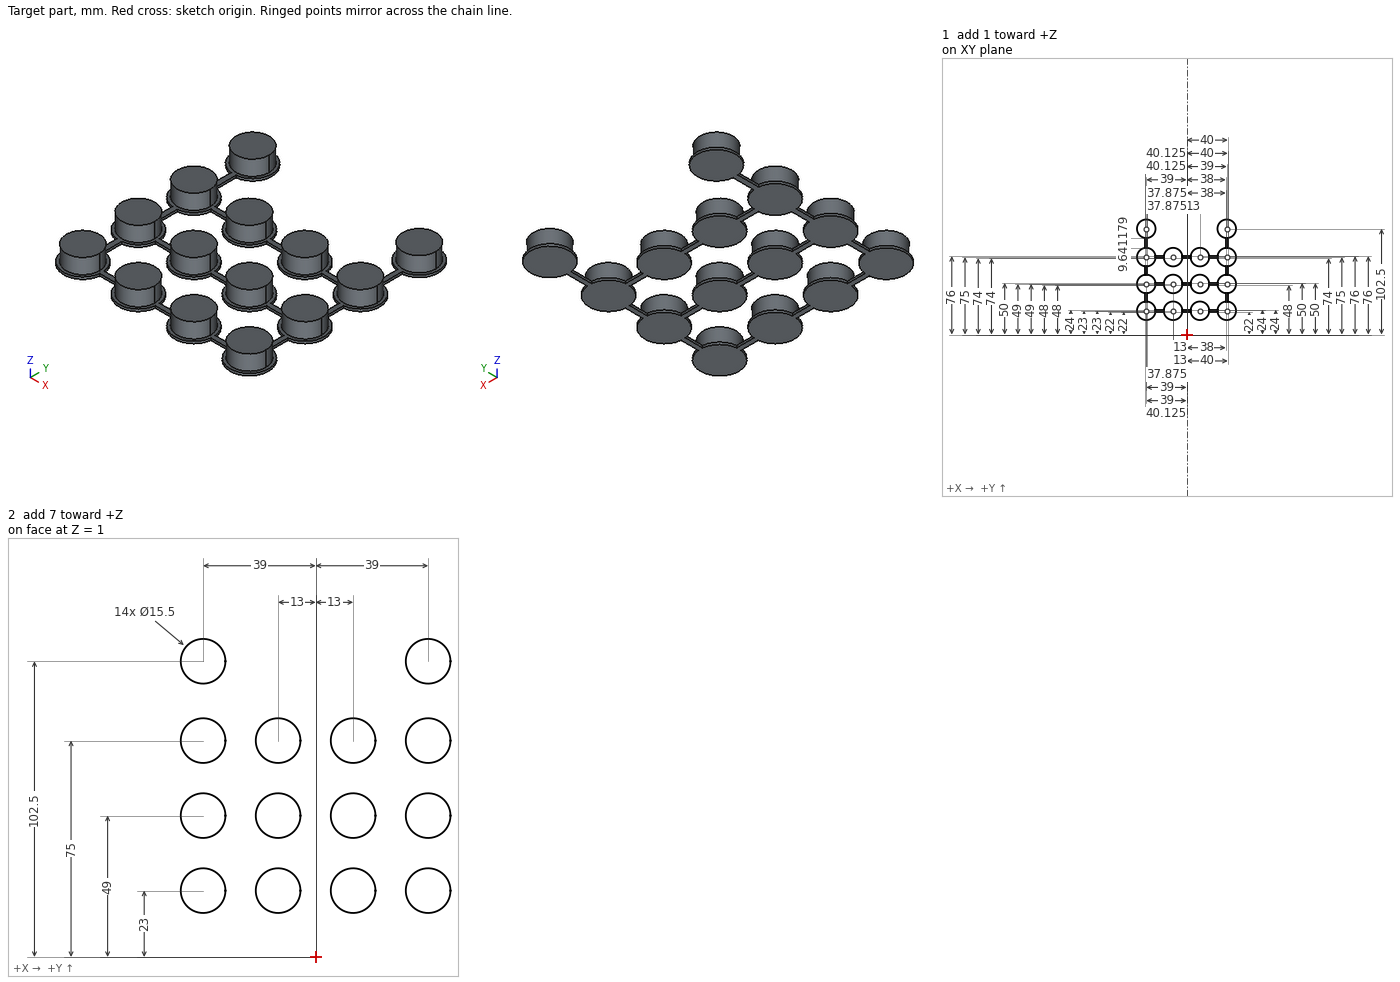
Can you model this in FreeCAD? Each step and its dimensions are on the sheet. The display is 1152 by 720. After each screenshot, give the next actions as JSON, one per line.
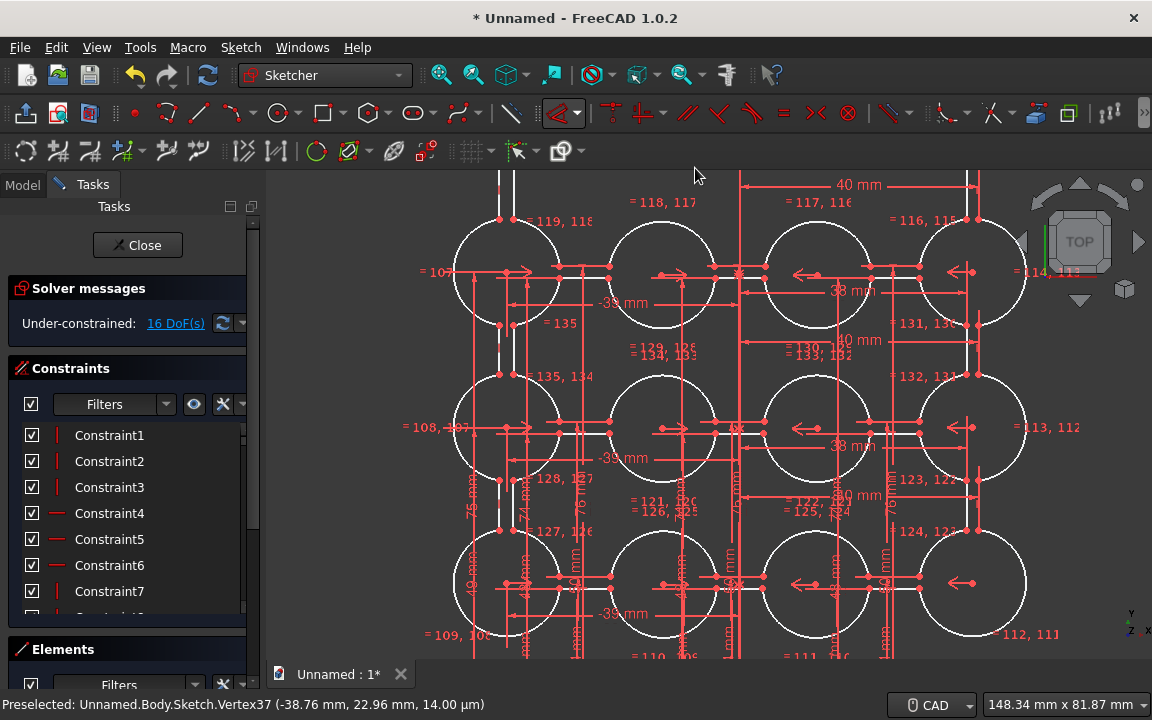
{"action": "left_click", "coordinate": [507, 583]}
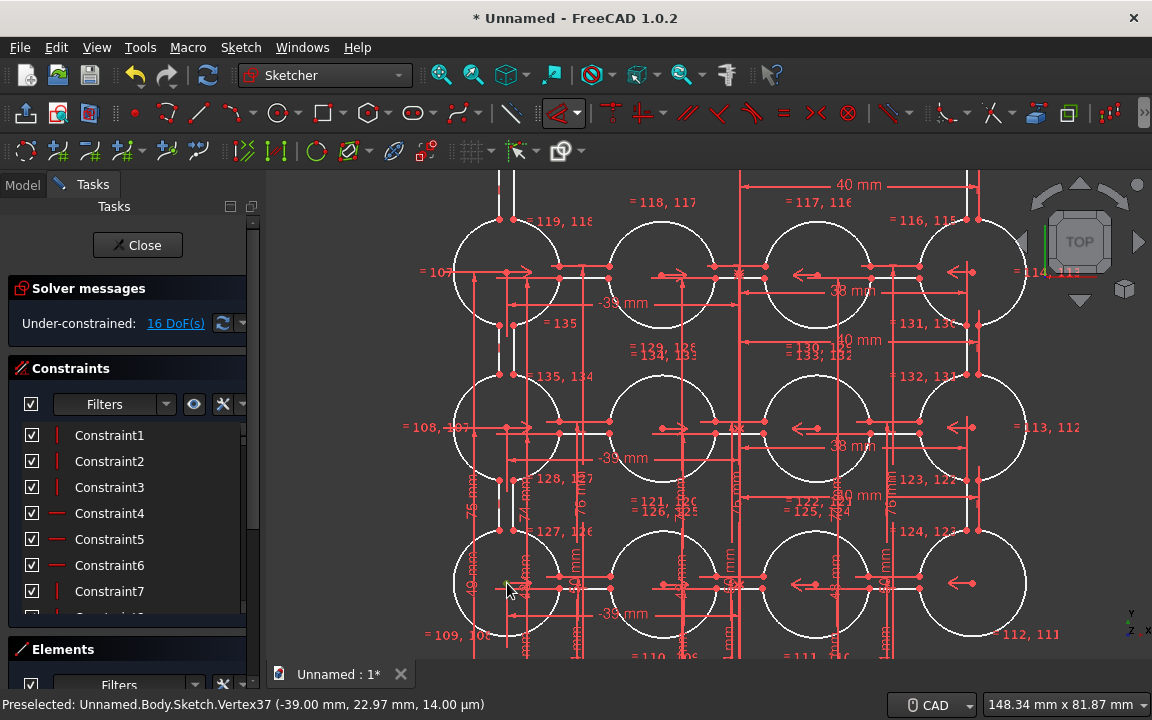
{"action": "key", "text": "i"}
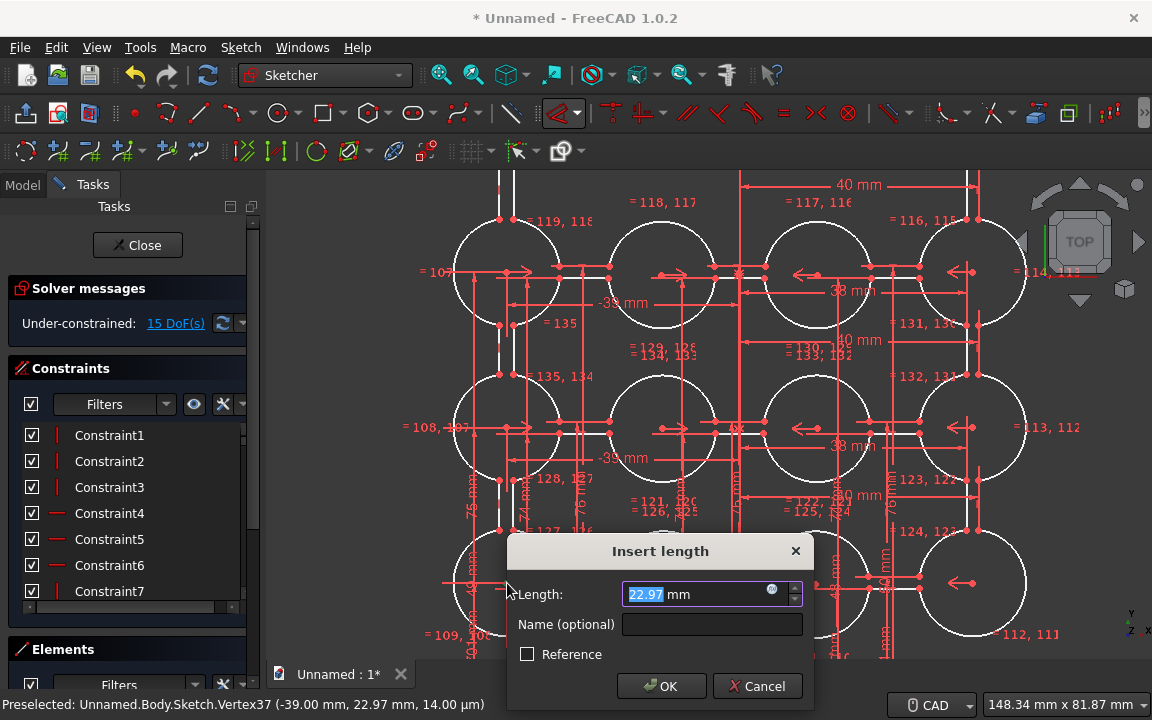
{"action": "type", "text": "23"}
{"action": "key", "text": "Return"}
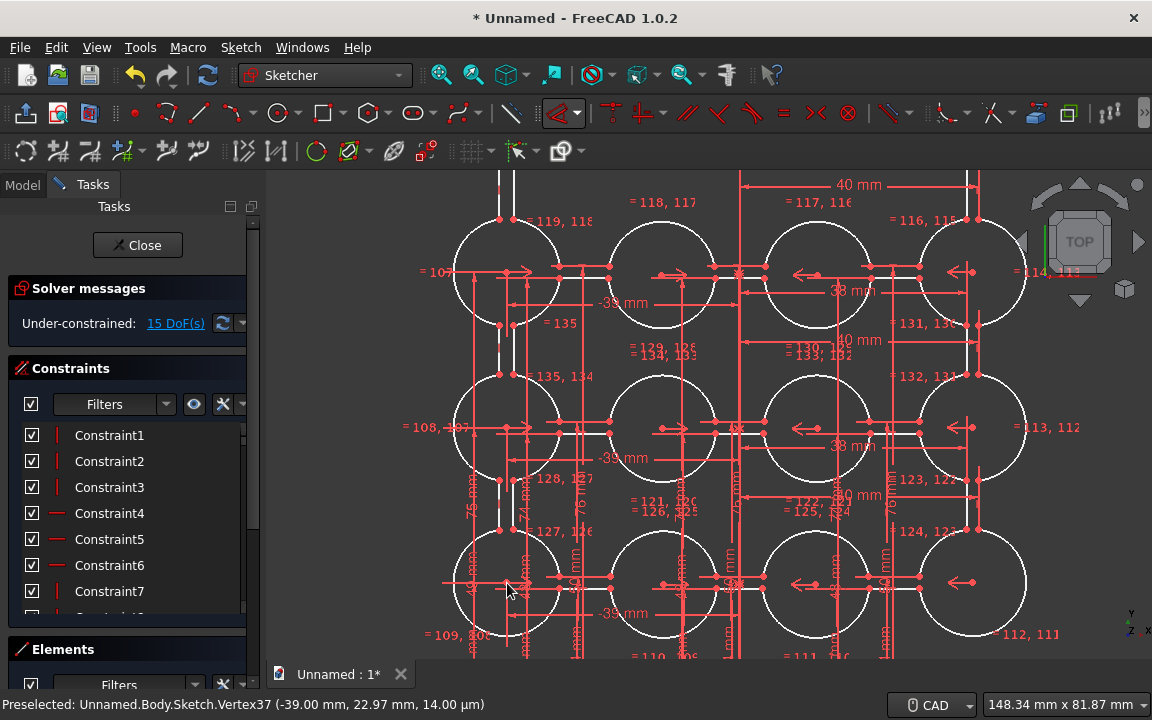
{"action": "left_click", "coordinate": [664, 585]}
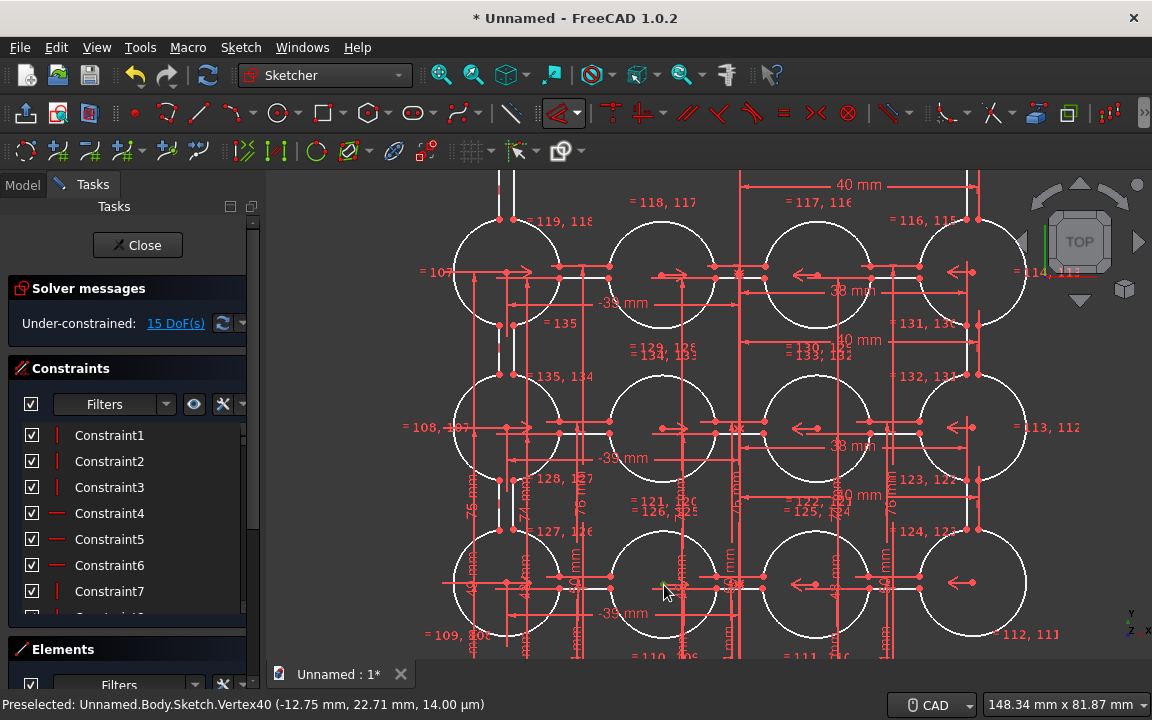
{"action": "key", "text": "l"}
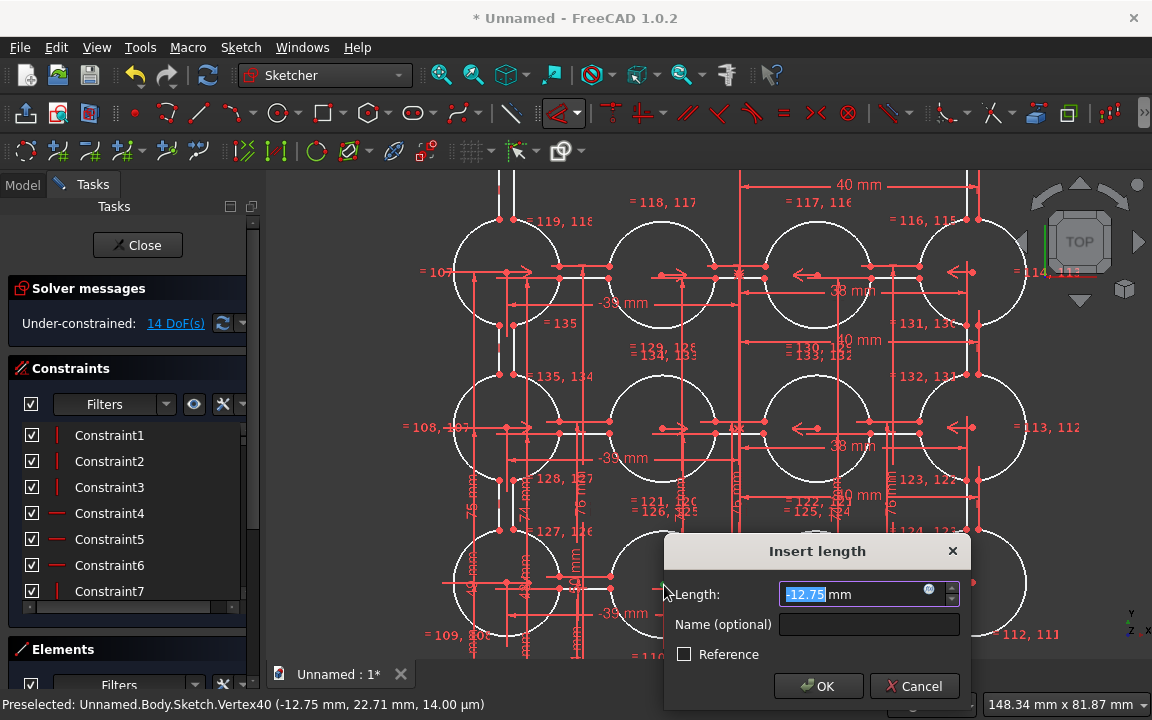
{"action": "type", "text": "-13"}
{"action": "key", "text": "Return"}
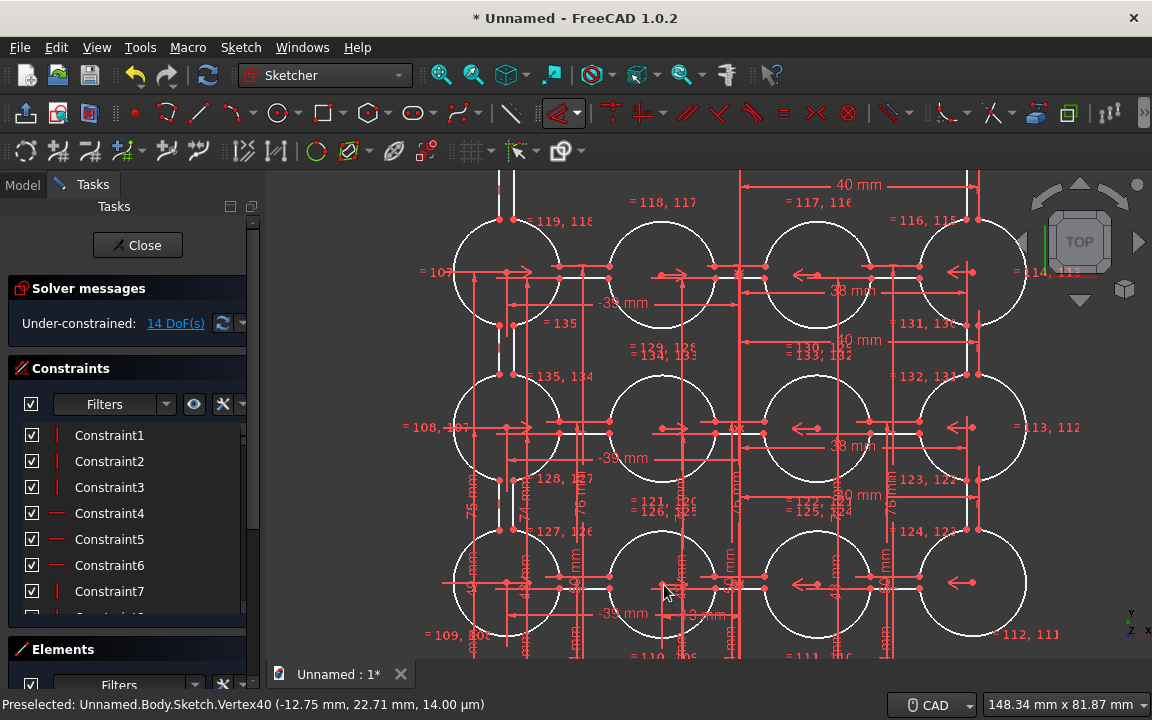
{"action": "left_click", "coordinate": [662, 585]}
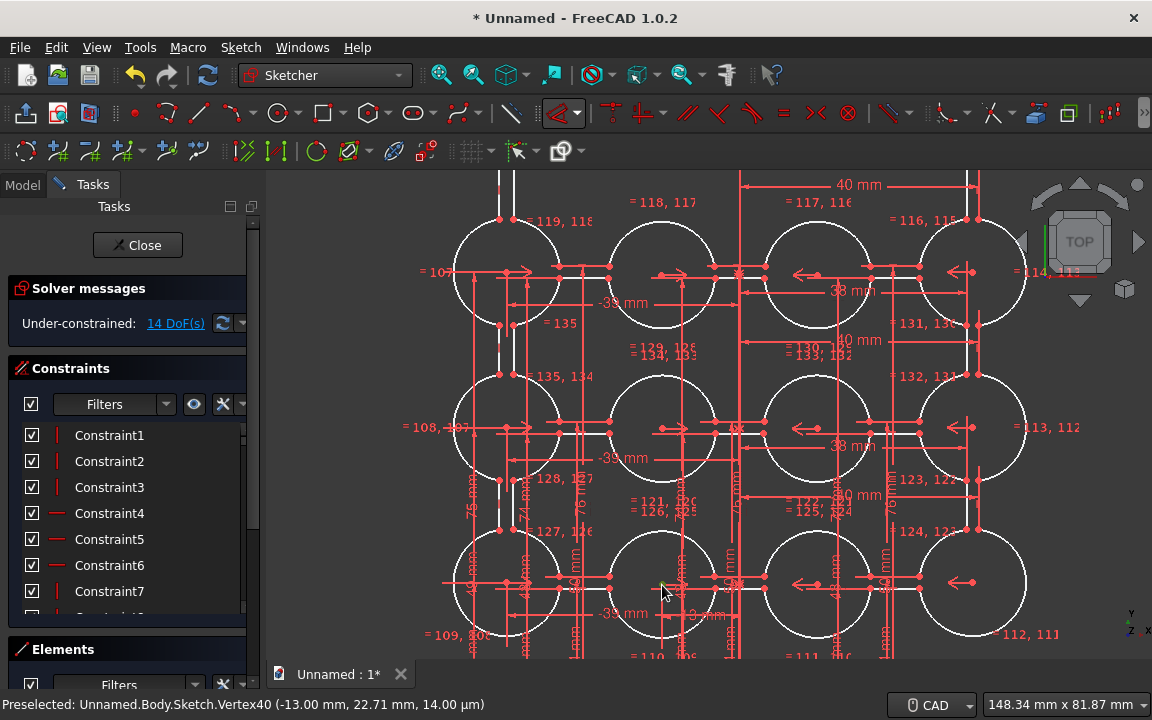
{"action": "key", "text": "i"}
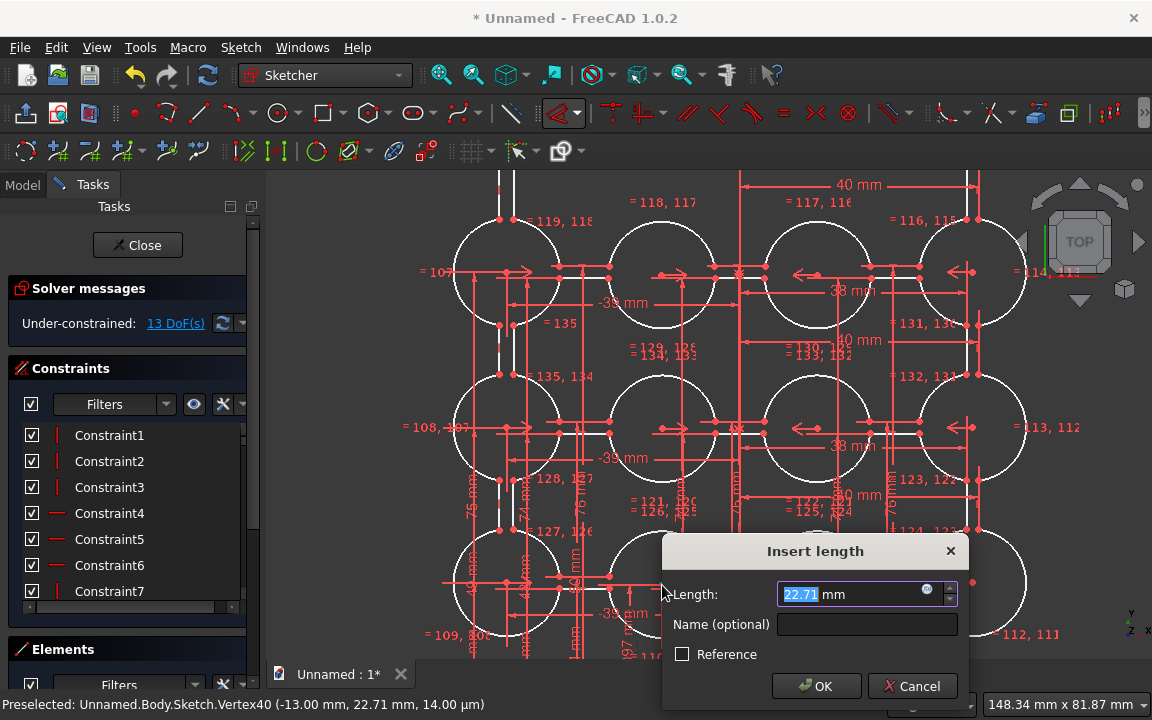
{"action": "type", "text": "23"}
{"action": "key", "text": "Return"}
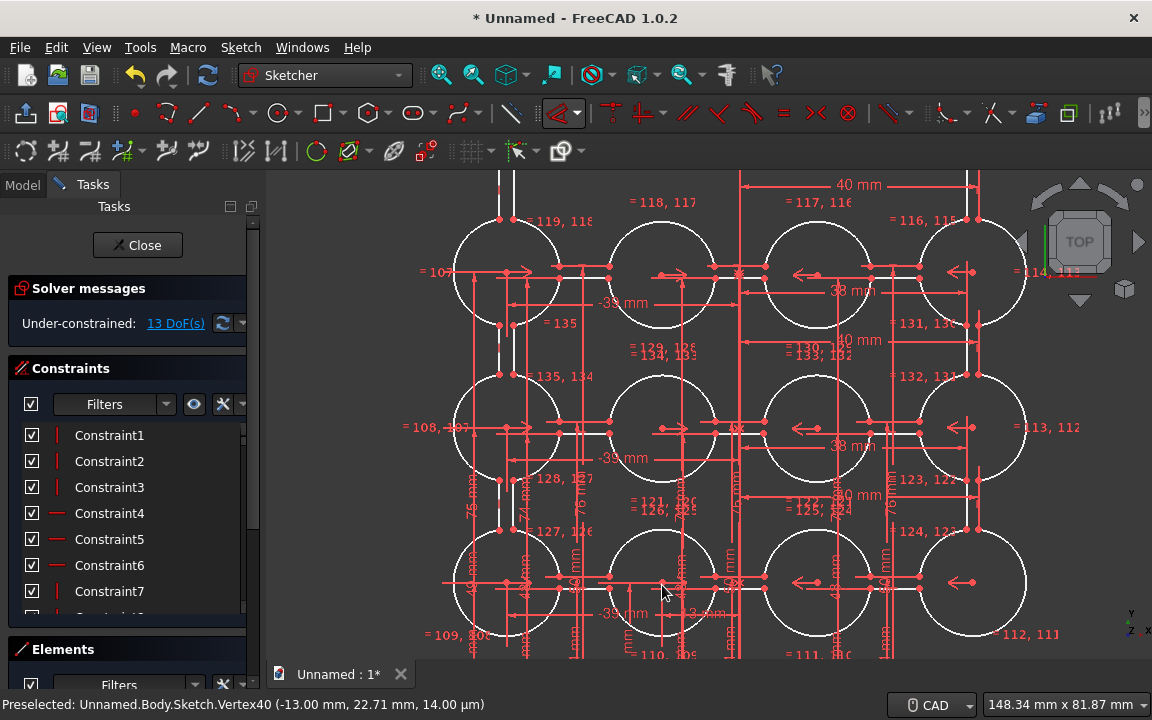
{"action": "scroll", "coordinate": [559, 437], "scroll_direction": "down", "scroll_amount": 4}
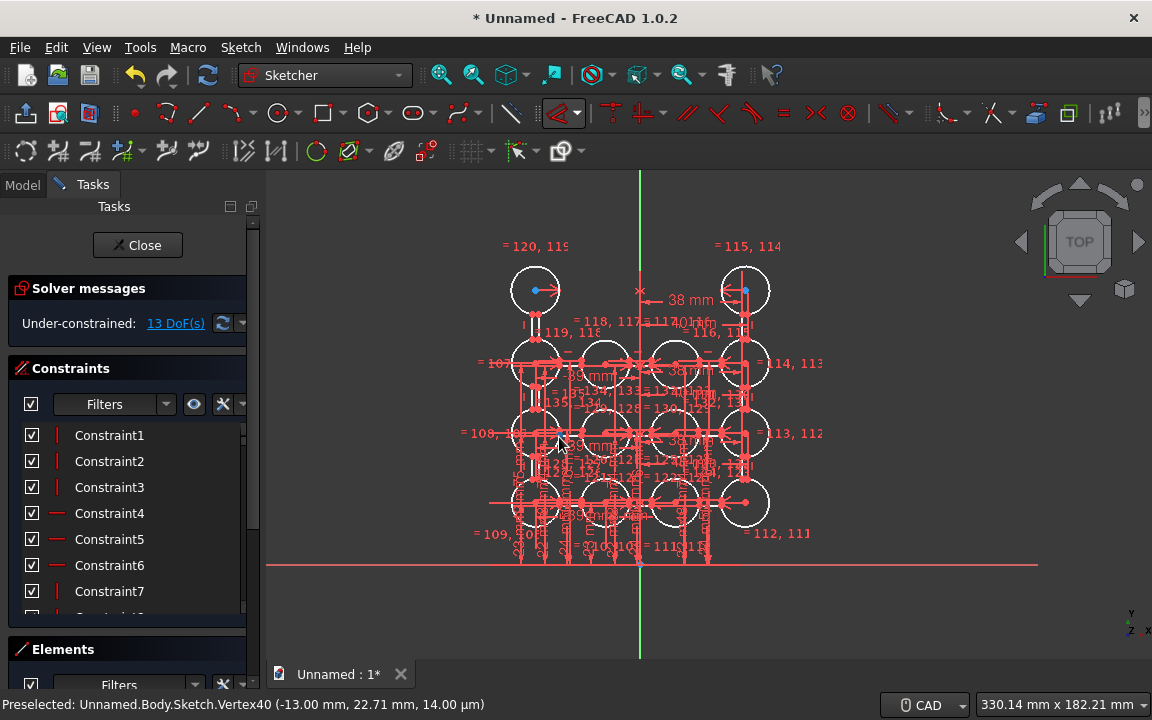
{"action": "left_click", "coordinate": [746, 290]}